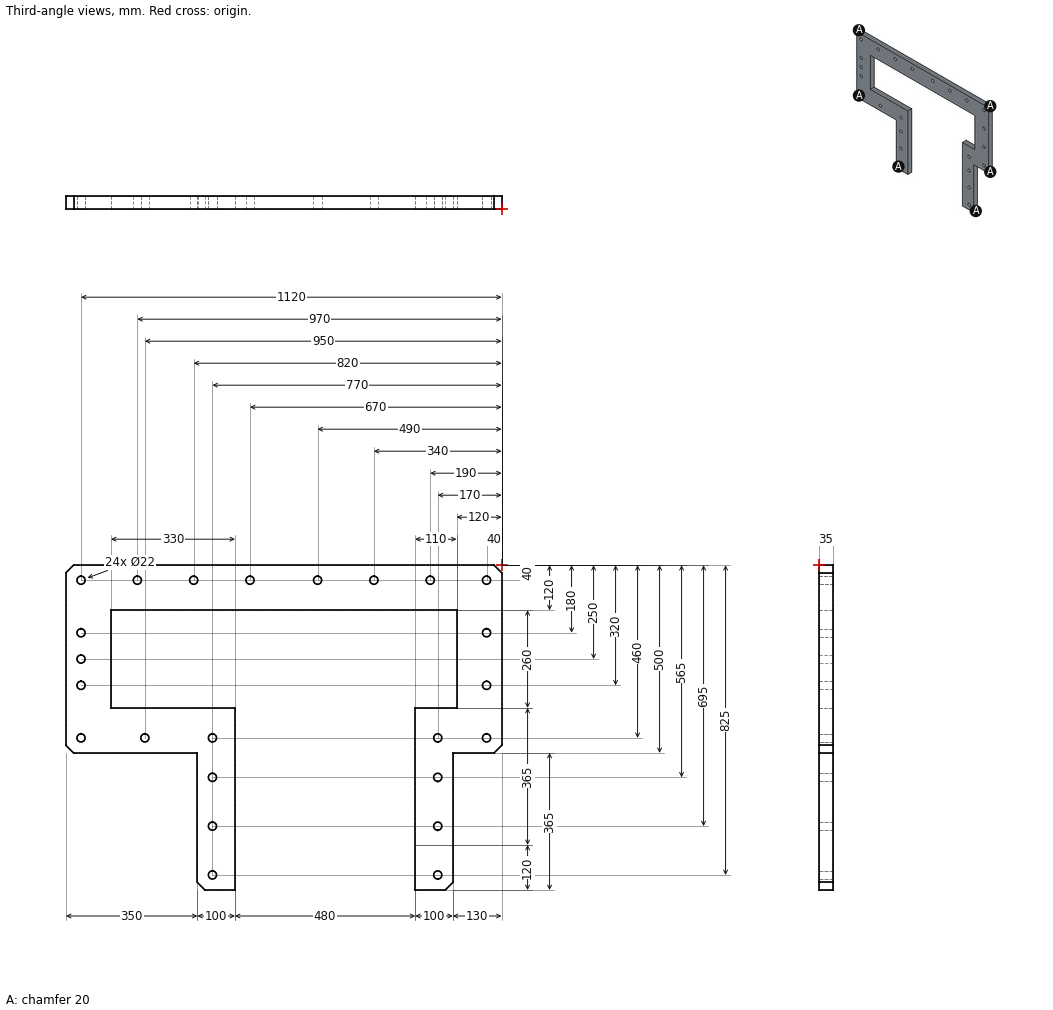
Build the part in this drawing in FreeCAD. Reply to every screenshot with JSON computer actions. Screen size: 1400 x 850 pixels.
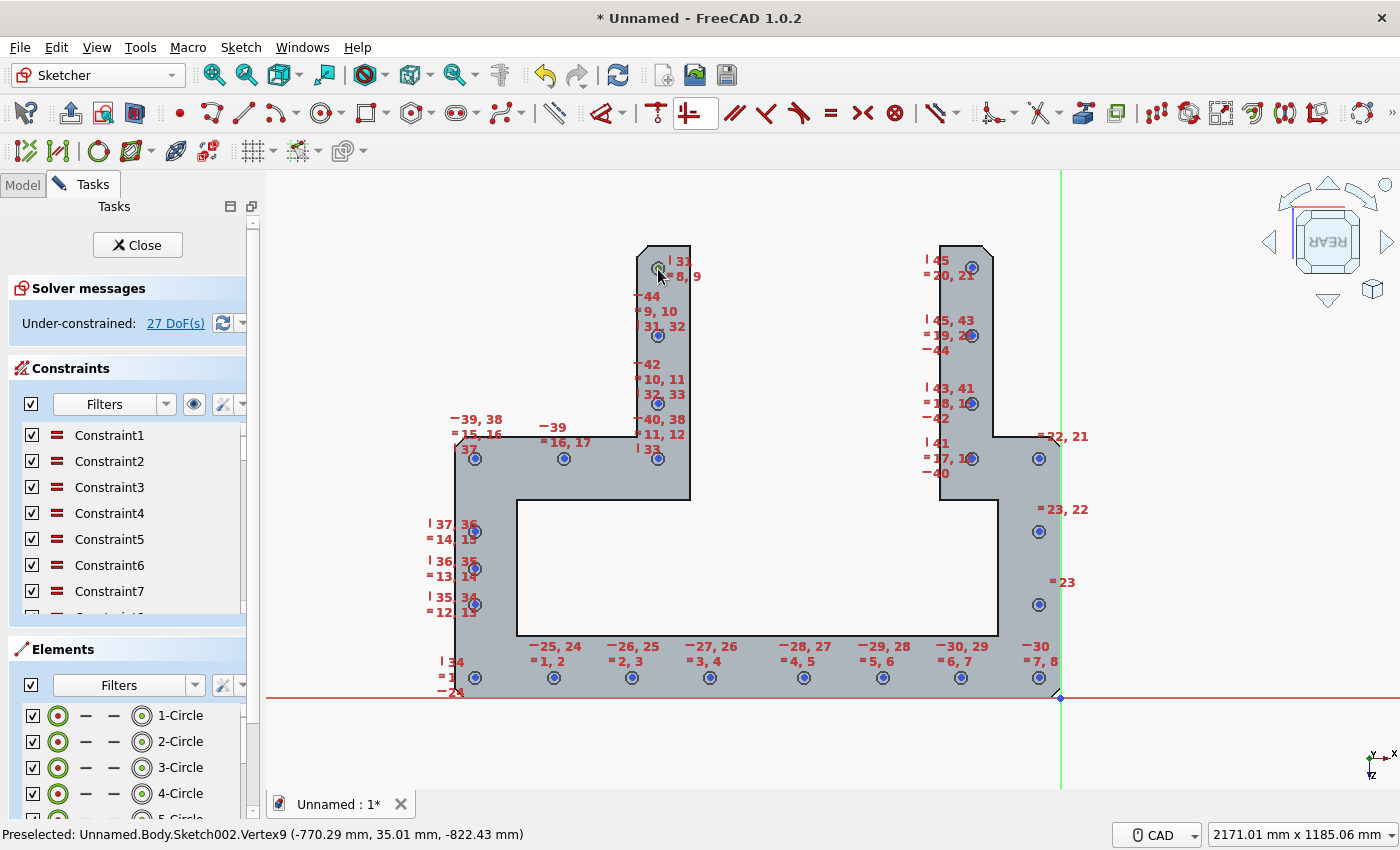
{"action": "left_click", "coordinate": [974, 270]}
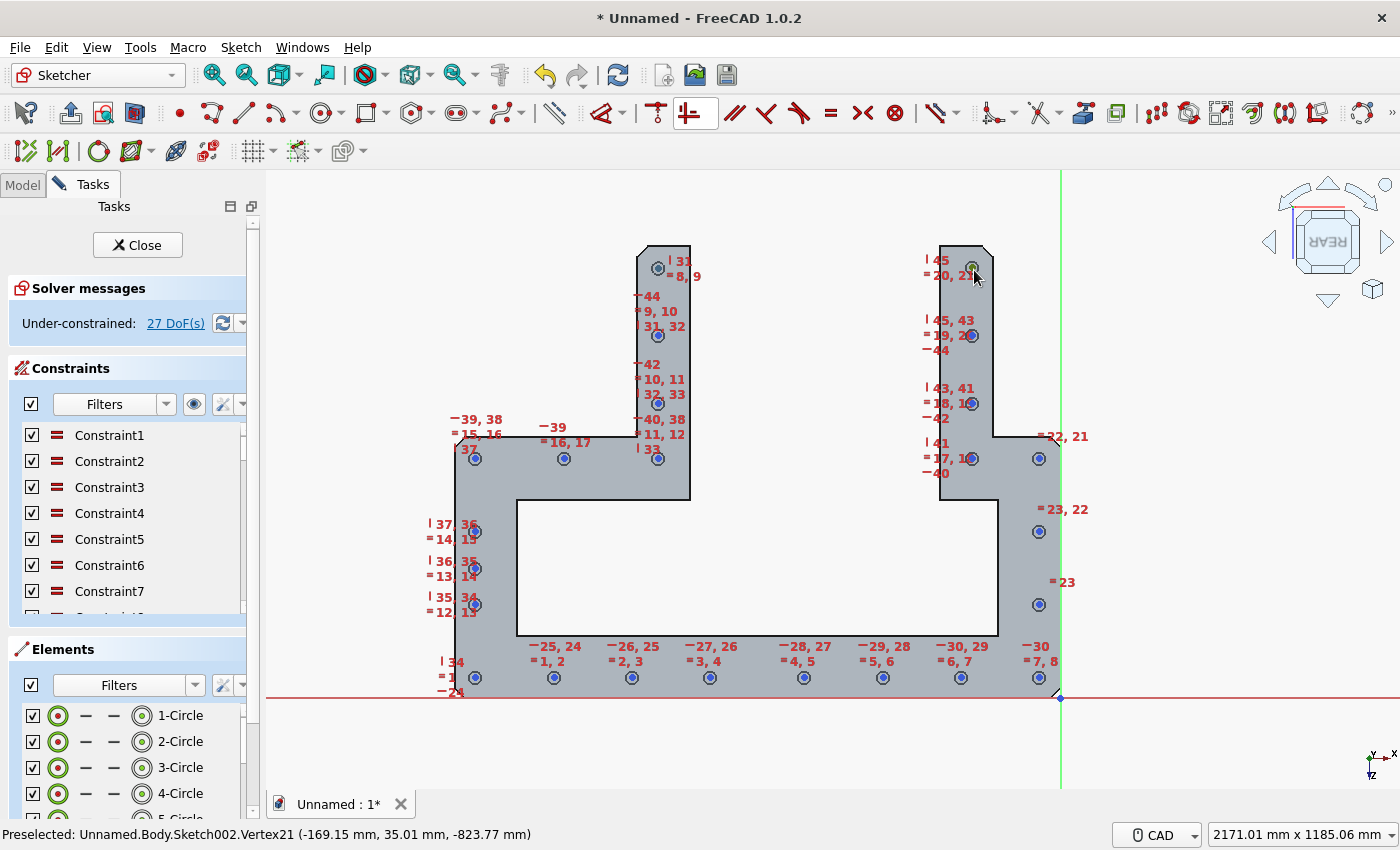
{"action": "key", "text": "h"}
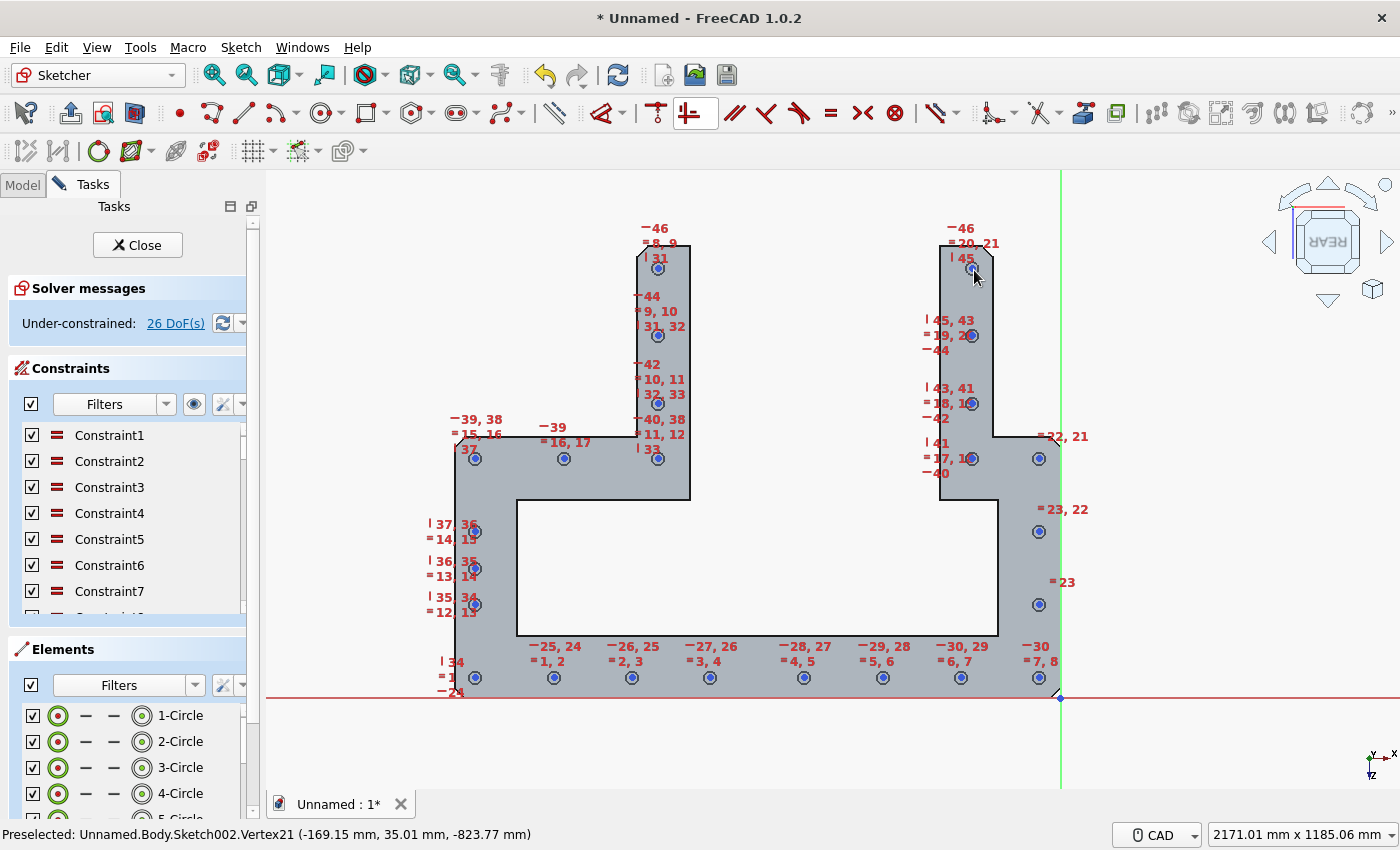
{"action": "left_click", "coordinate": [1039, 678]}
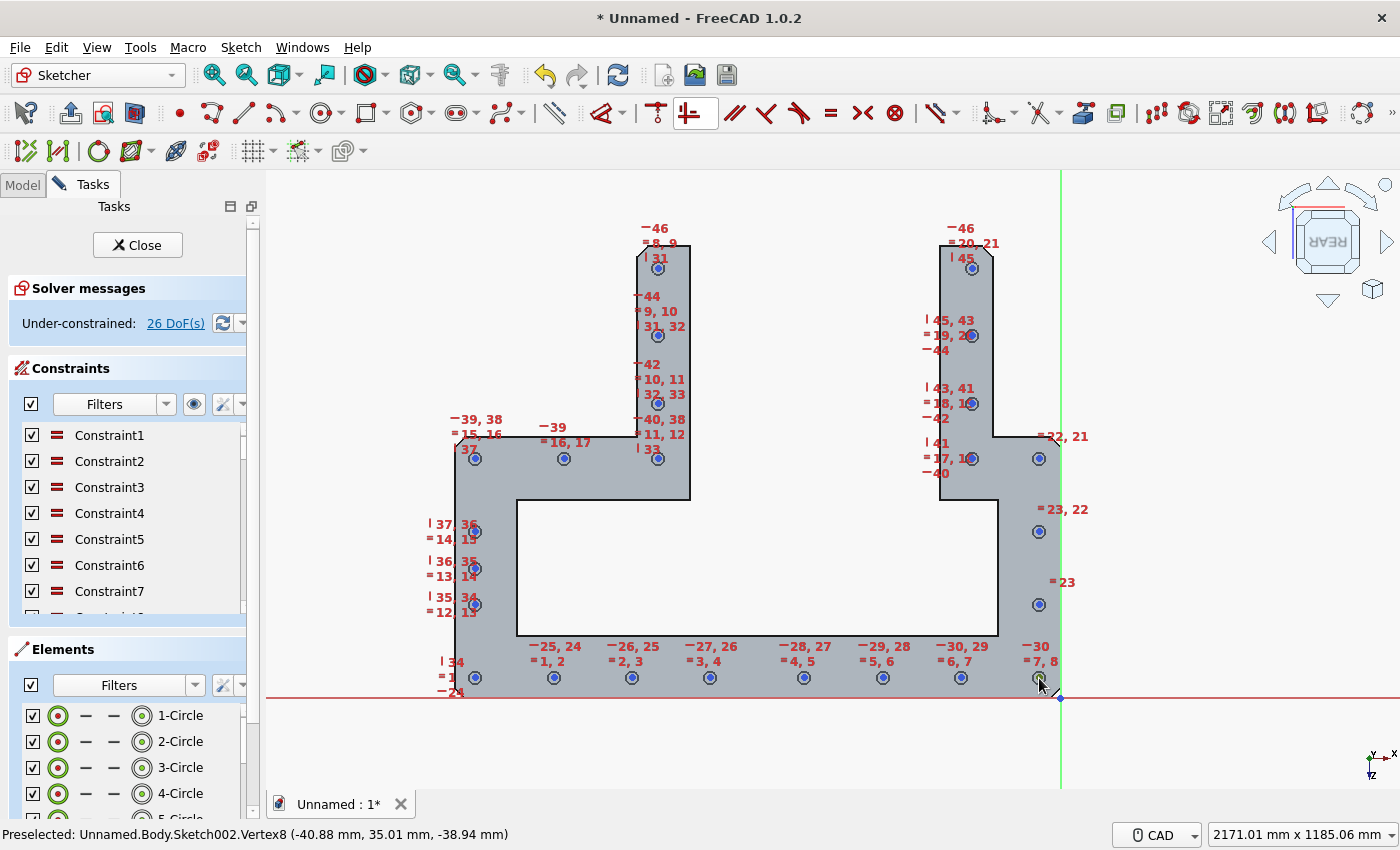
{"action": "left_click", "coordinate": [1039, 459]}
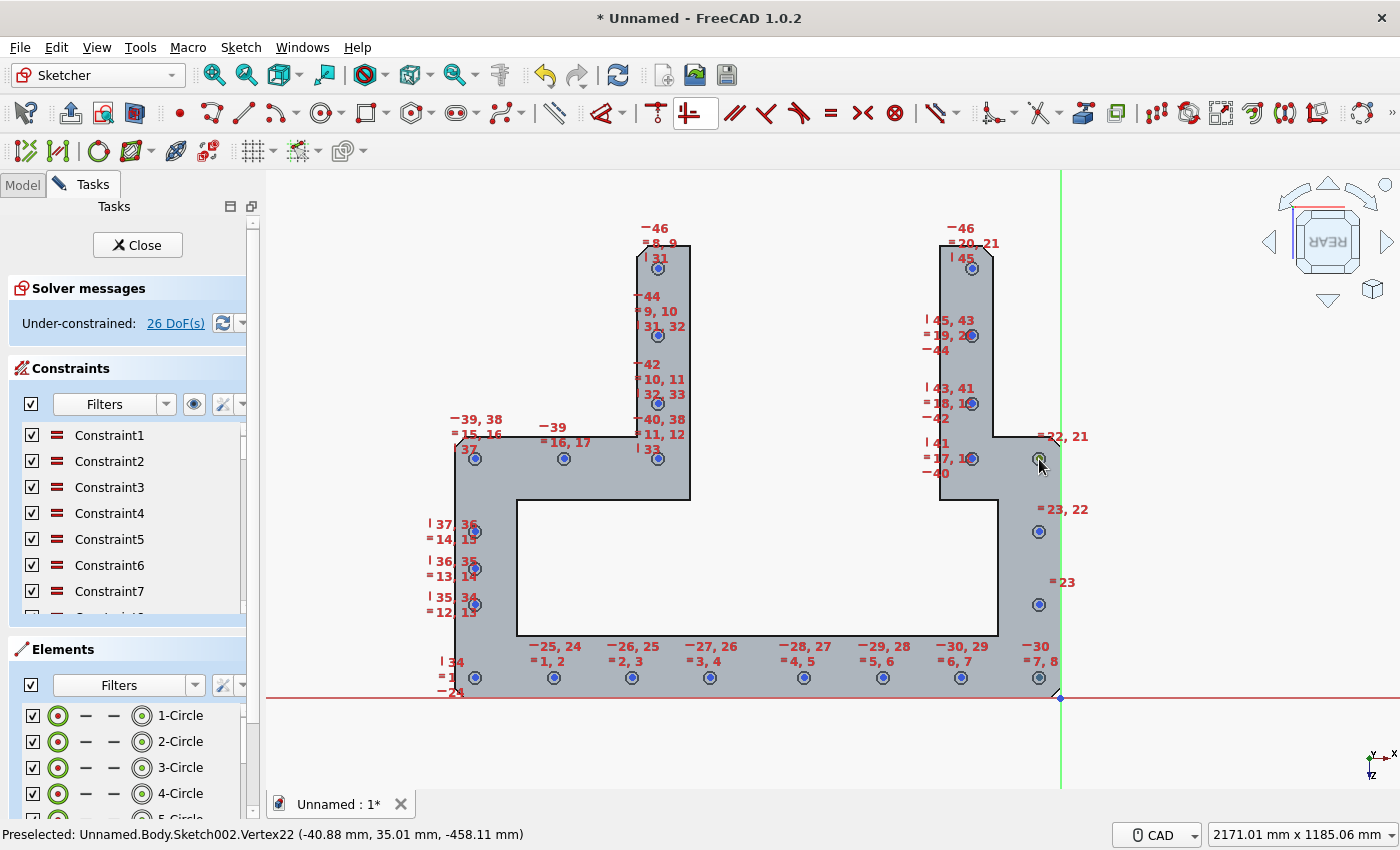
{"action": "key", "text": "v"}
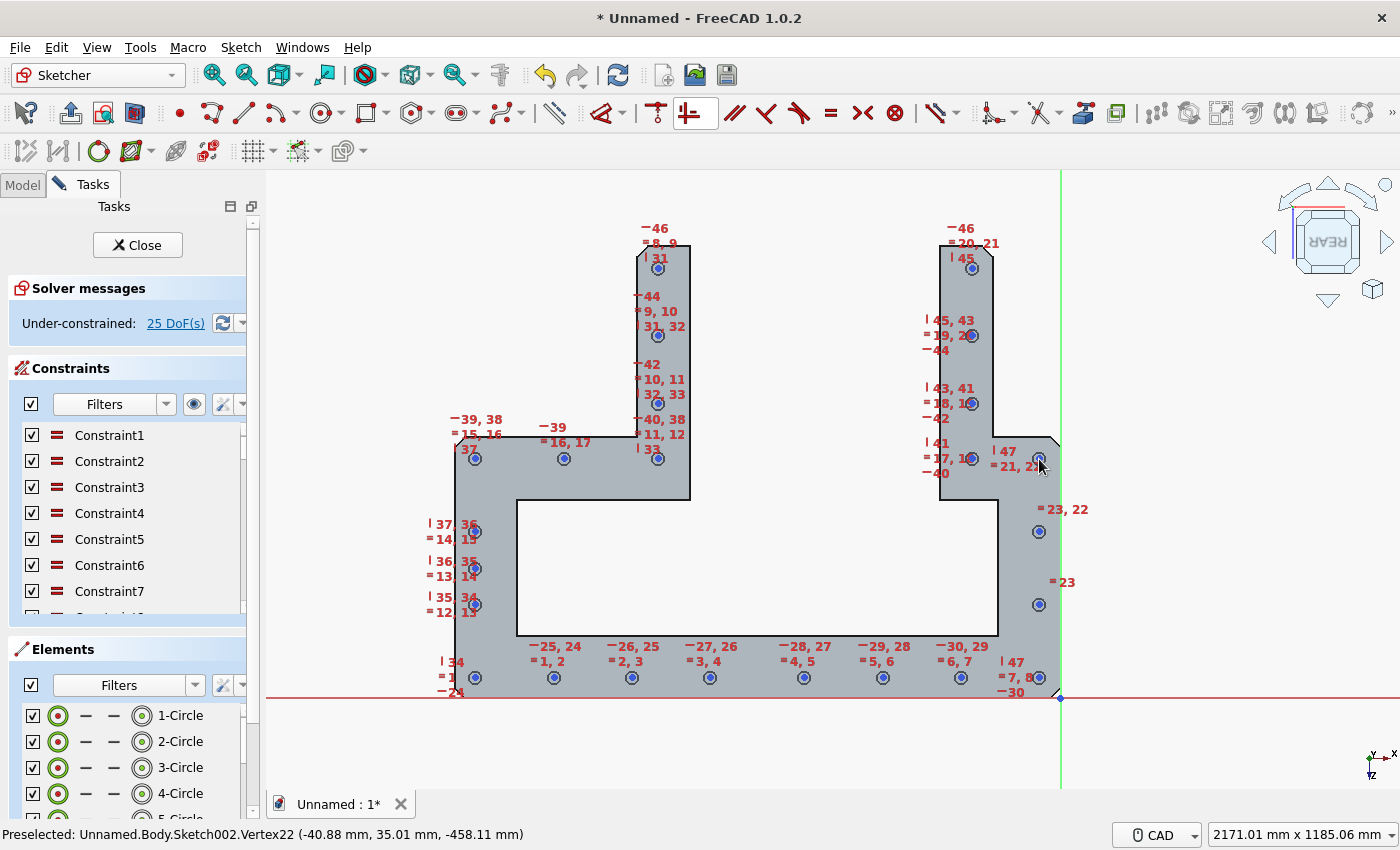
{"action": "left_click", "coordinate": [972, 459]}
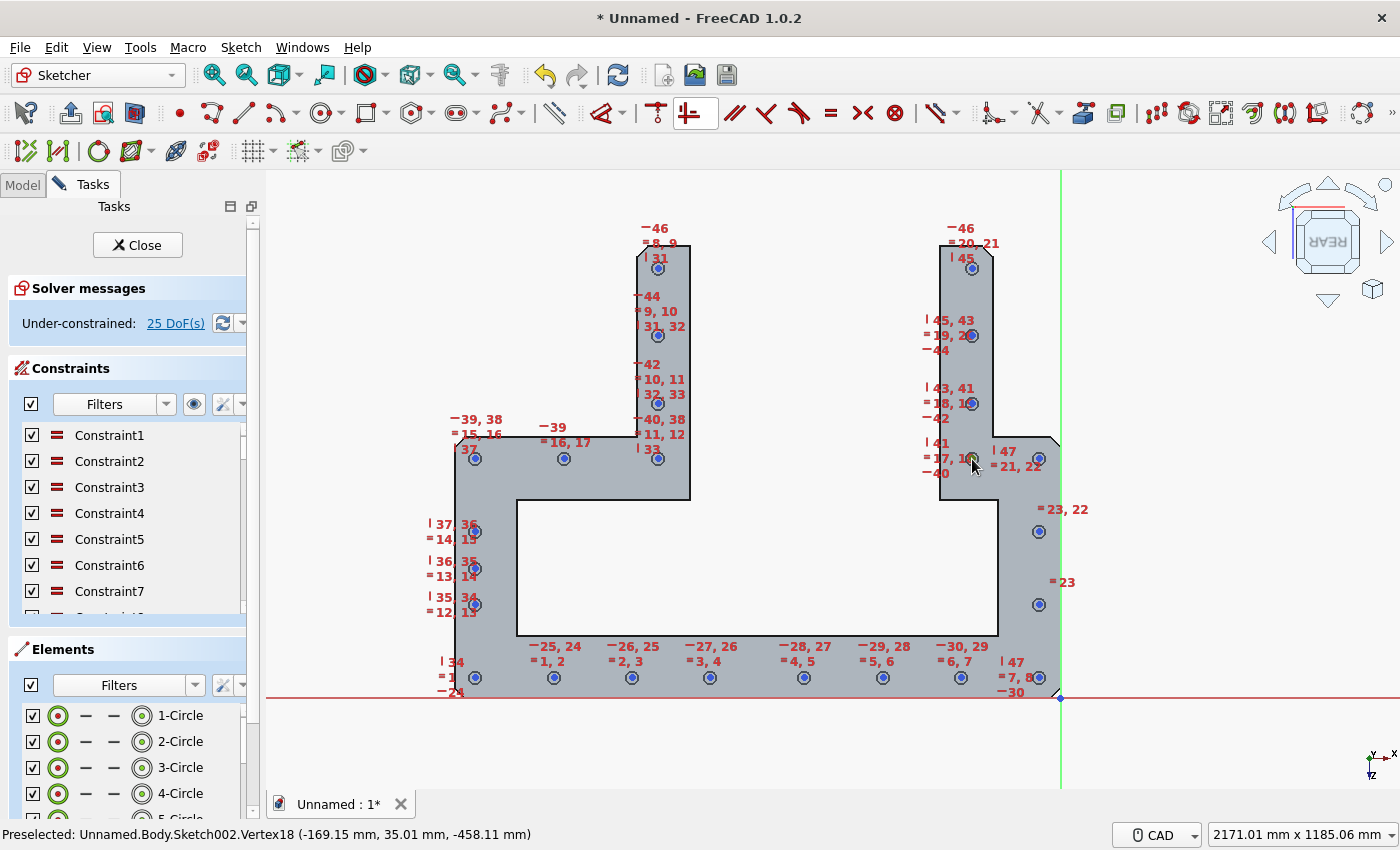
{"action": "left_click", "coordinate": [1041, 461]}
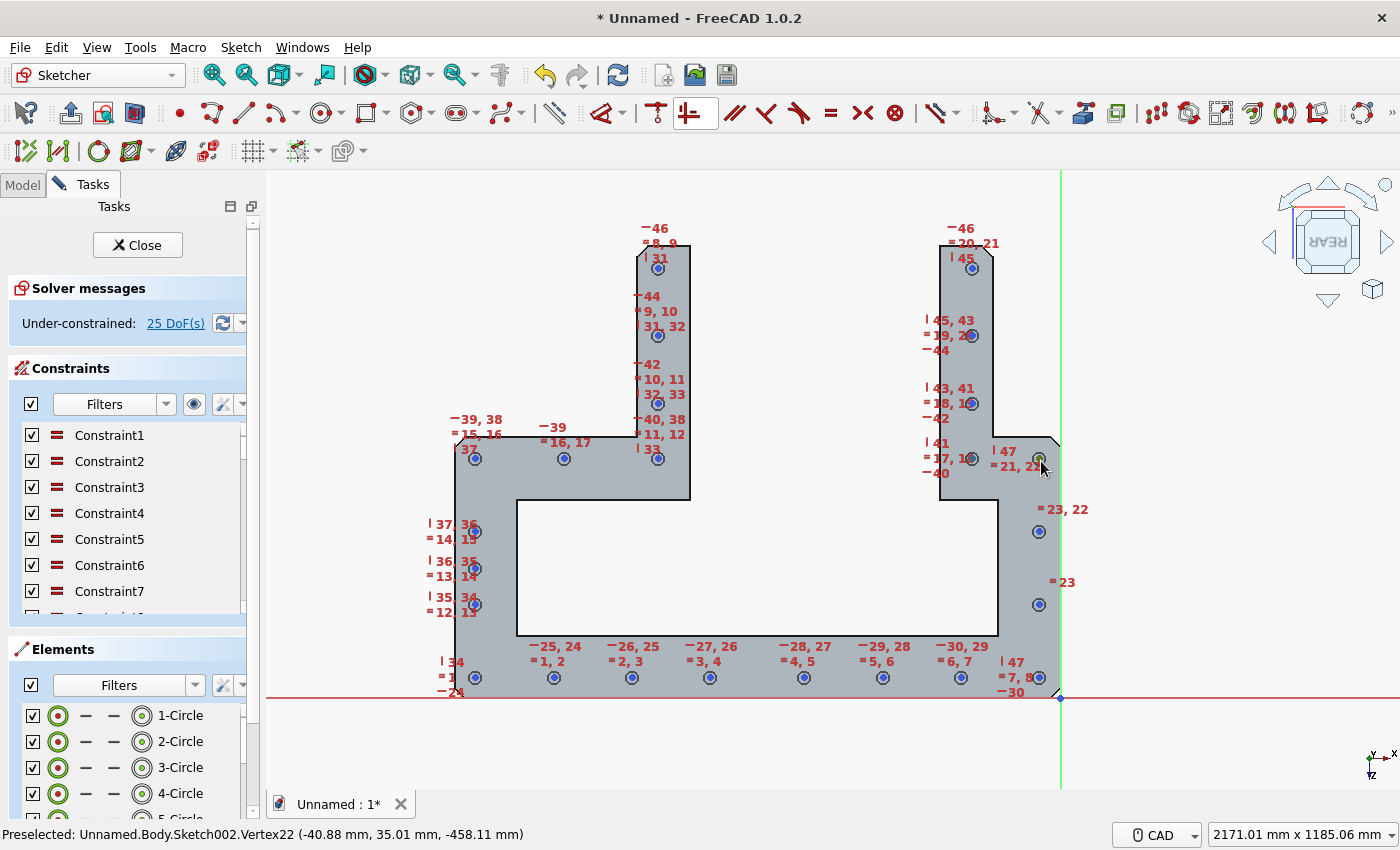
{"action": "key", "text": "h"}